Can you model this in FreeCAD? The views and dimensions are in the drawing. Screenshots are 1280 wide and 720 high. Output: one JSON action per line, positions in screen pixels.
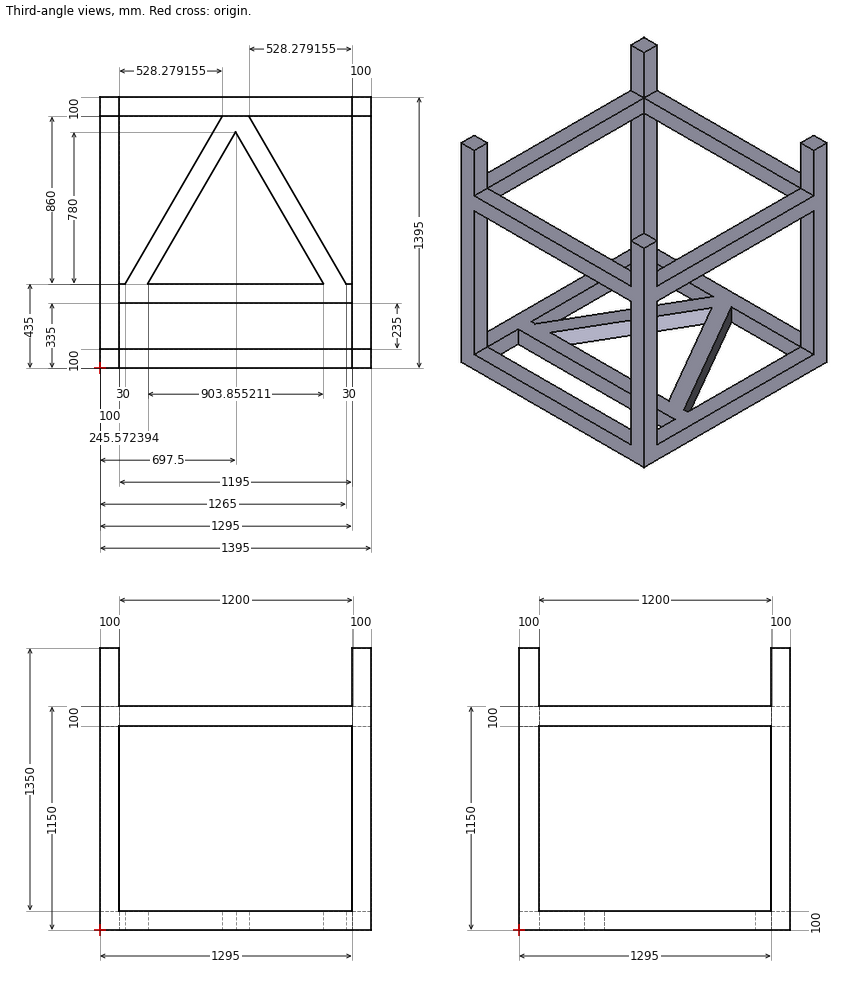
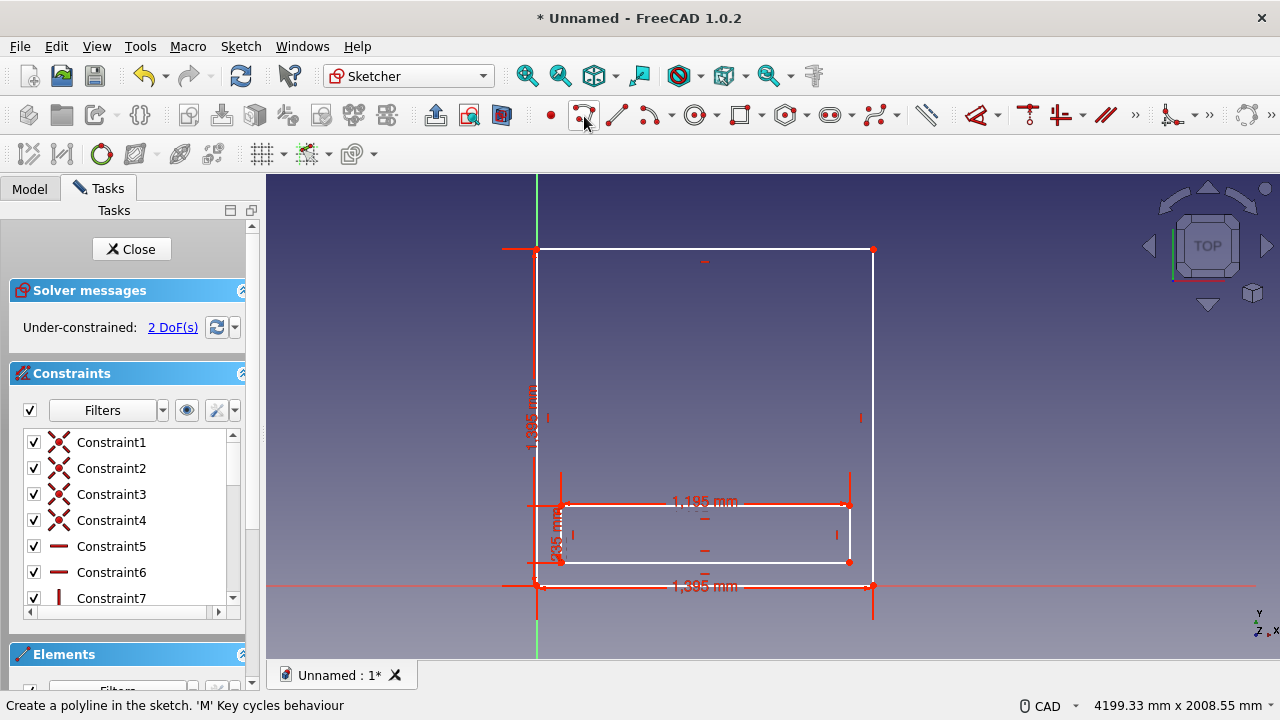
{"action": "left_click", "coordinate": [561, 481]}
{"action": "left_click", "coordinate": [561, 273]}
{"action": "left_click", "coordinate": [688, 273]}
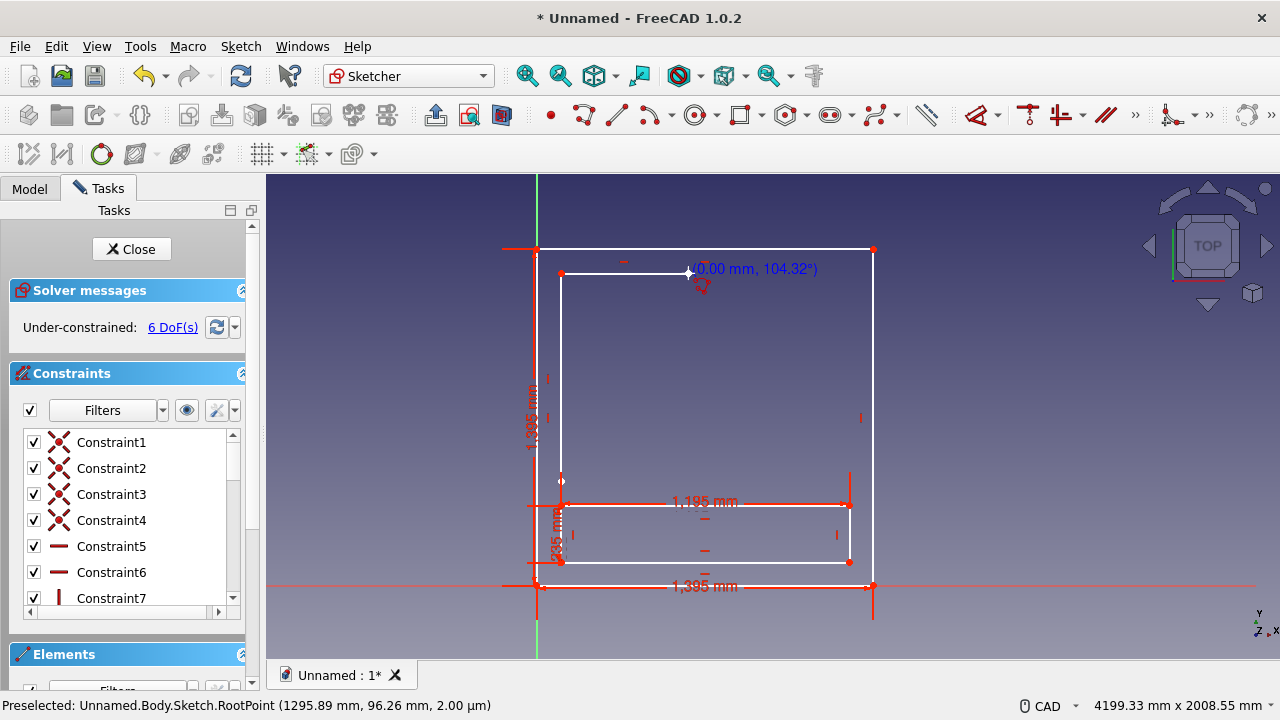
{"action": "scroll", "coordinate": [568, 481], "scroll_direction": "up", "scroll_amount": 4}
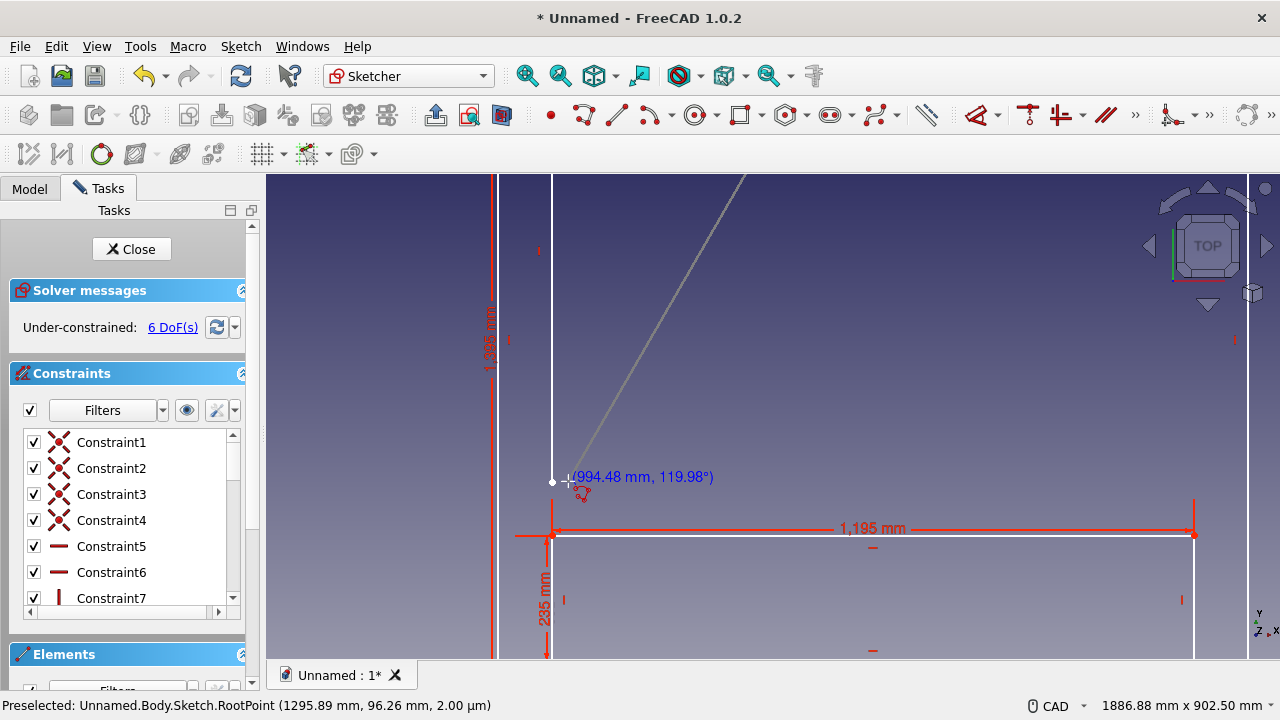
{"action": "left_click", "coordinate": [568, 480]}
{"action": "left_click", "coordinate": [552, 482]}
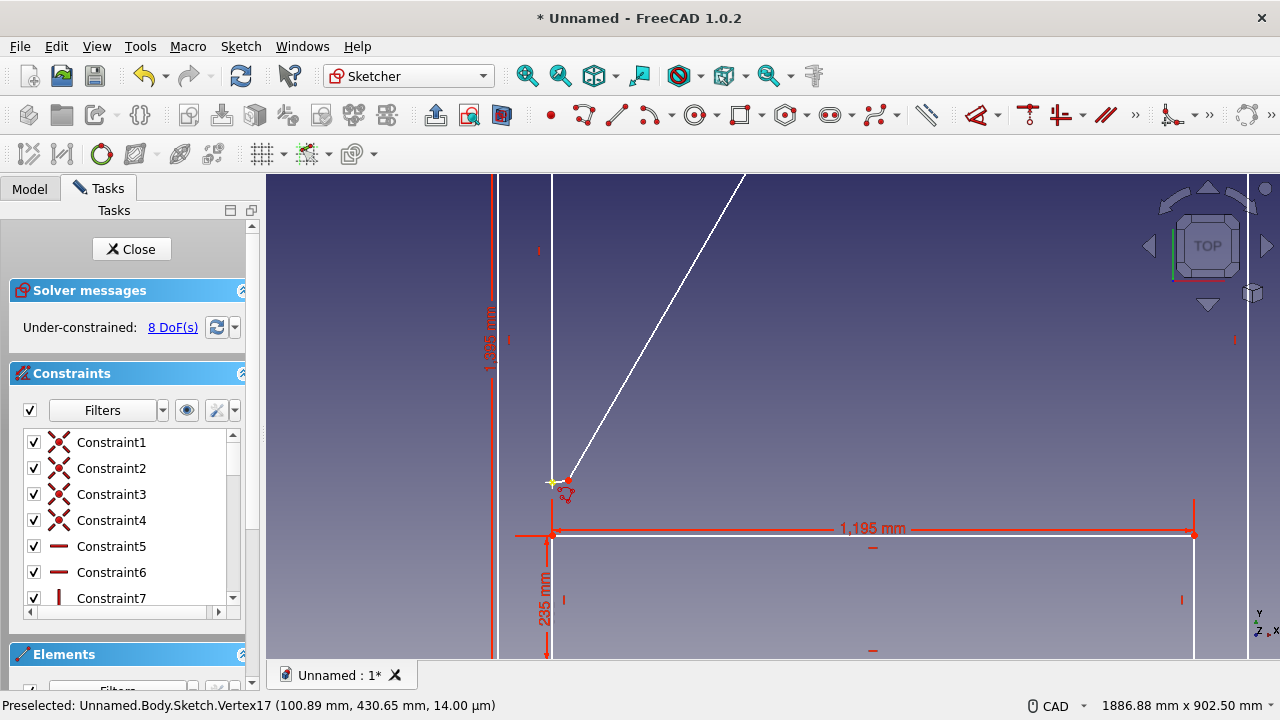
{"action": "left_click", "coordinate": [630, 480]}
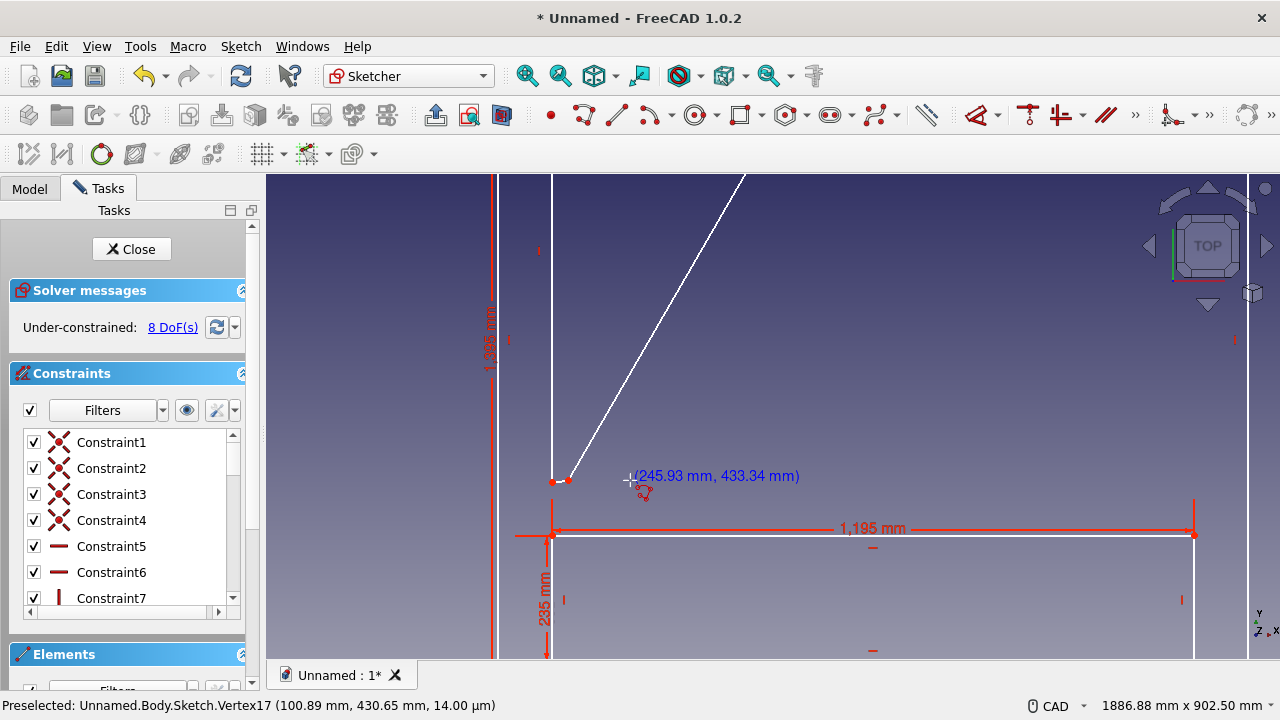
{"action": "scroll", "coordinate": [607, 462], "scroll_direction": "down", "scroll_amount": 5}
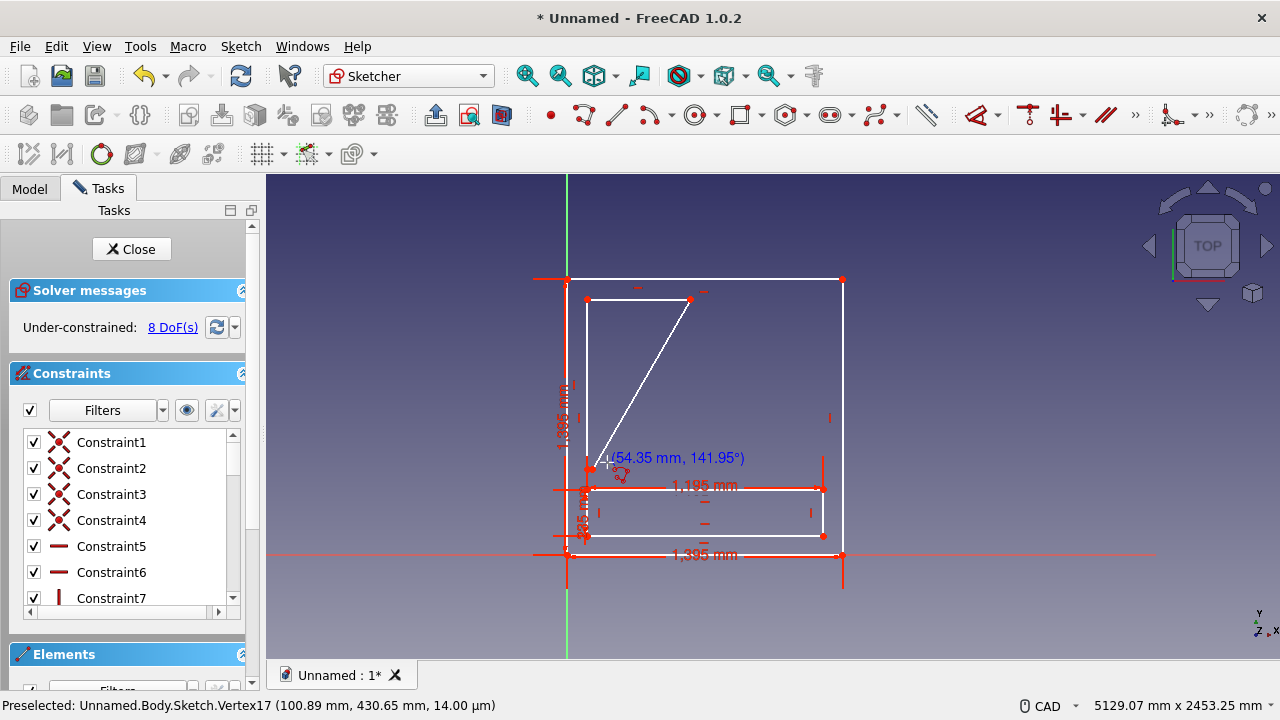
{"action": "left_click", "coordinate": [705, 315]}
{"action": "left_click", "coordinate": [794, 469]}
{"action": "left_click", "coordinate": [616, 469]}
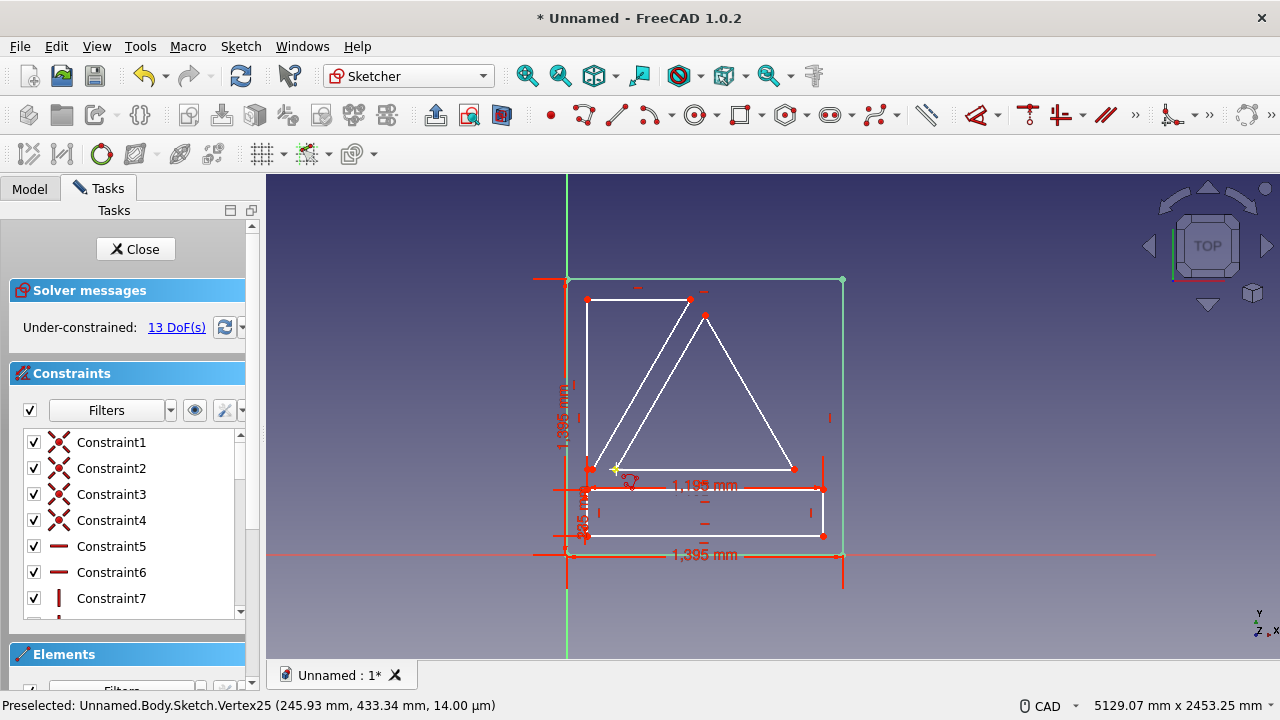
{"action": "left_click", "coordinate": [817, 469]}
{"action": "left_click", "coordinate": [719, 299]}
{"action": "left_click", "coordinate": [823, 299]}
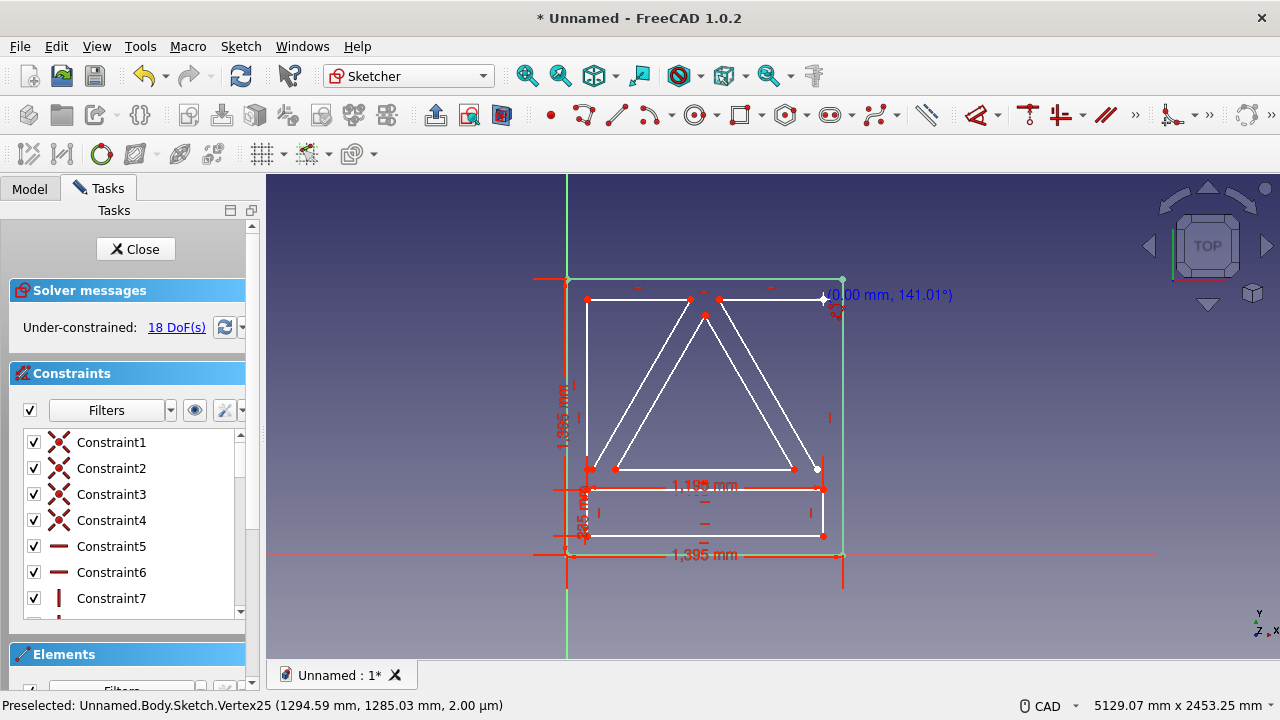
{"action": "scroll", "coordinate": [823, 469], "scroll_direction": "up", "scroll_amount": 5}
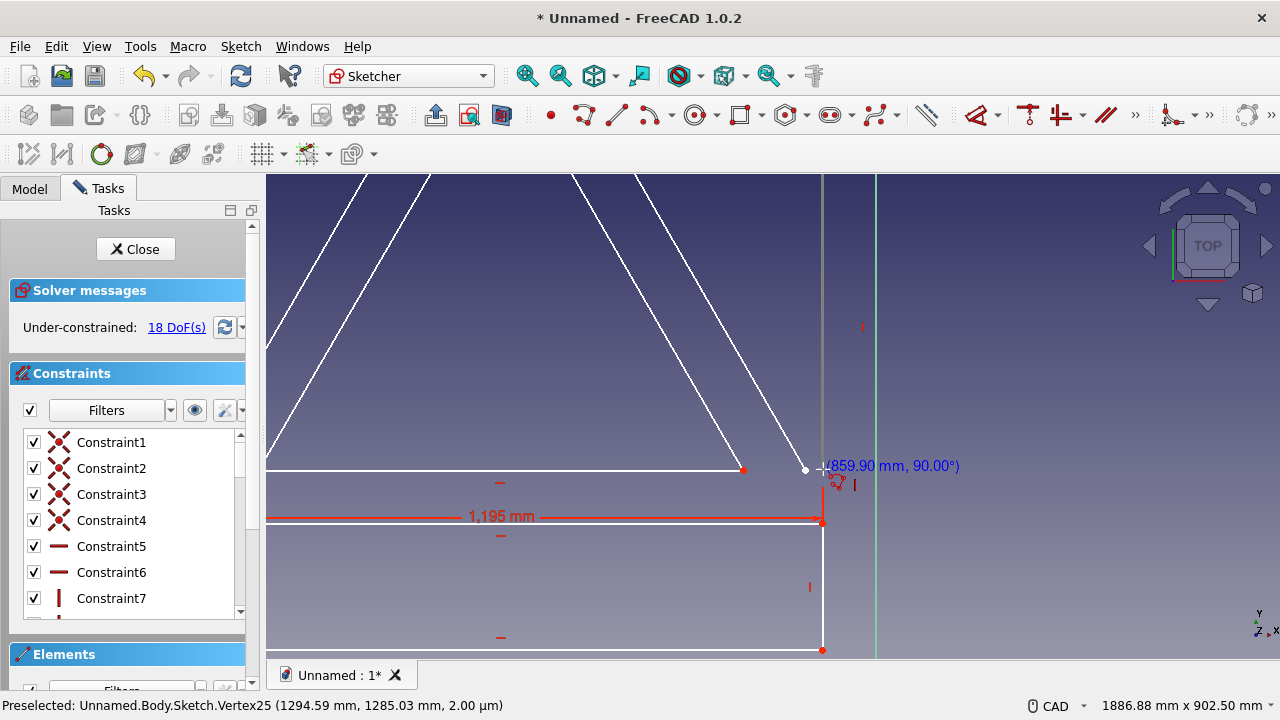
{"action": "left_click", "coordinate": [822, 468]}
{"action": "left_click", "coordinate": [806, 471]}
{"action": "key", "text": "Escape"}
{"action": "key", "text": "Escape"}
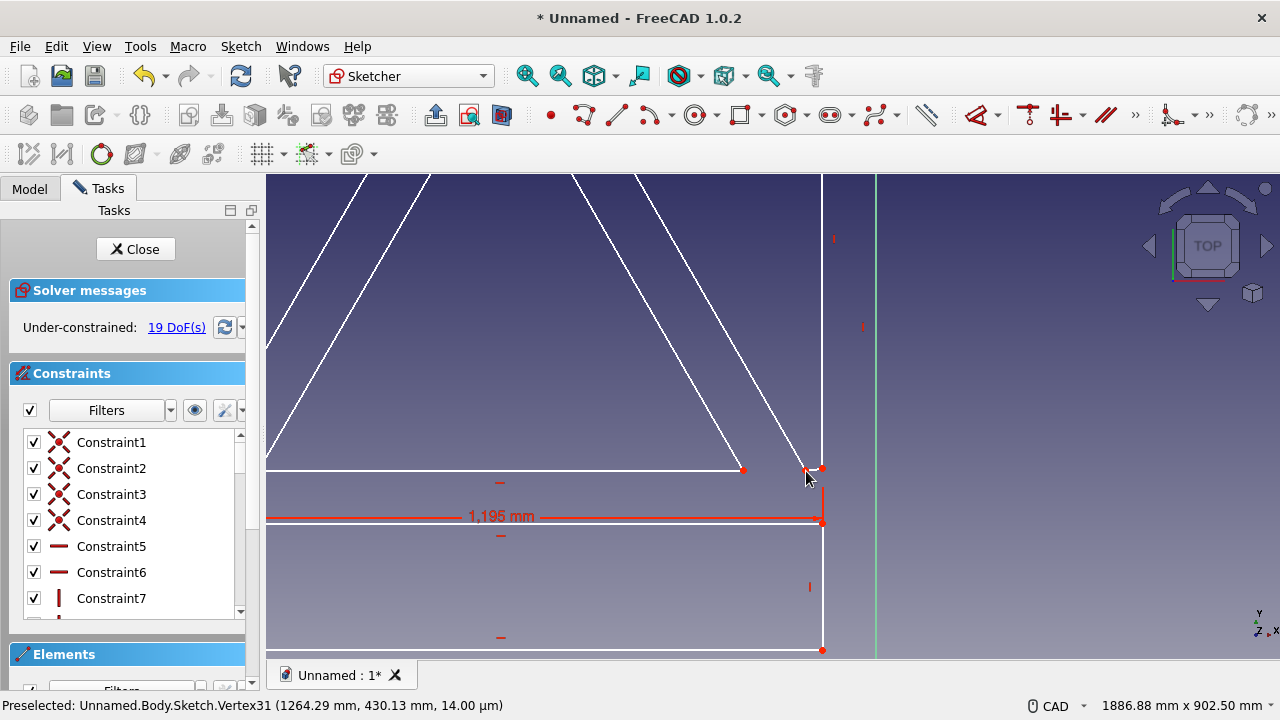
{"action": "scroll", "coordinate": [823, 469], "scroll_direction": "down", "scroll_amount": 5}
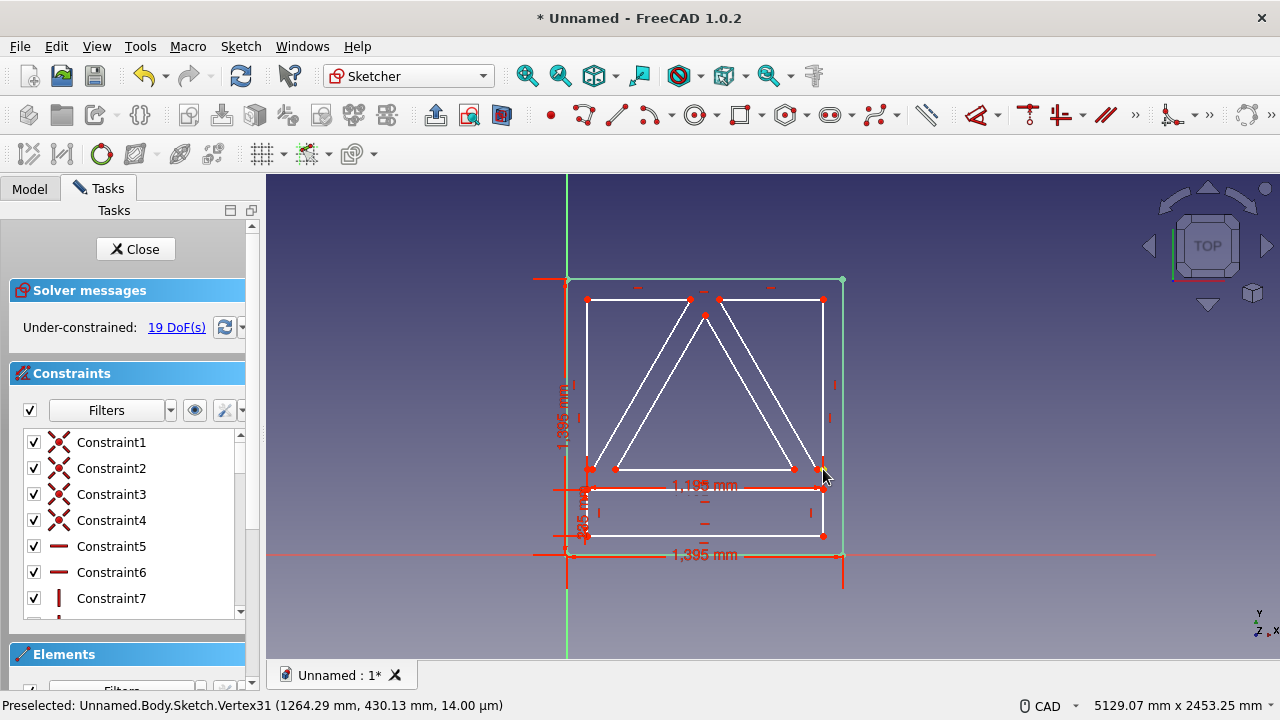
{"action": "scroll", "coordinate": [590, 470], "scroll_direction": "up", "scroll_amount": 8}